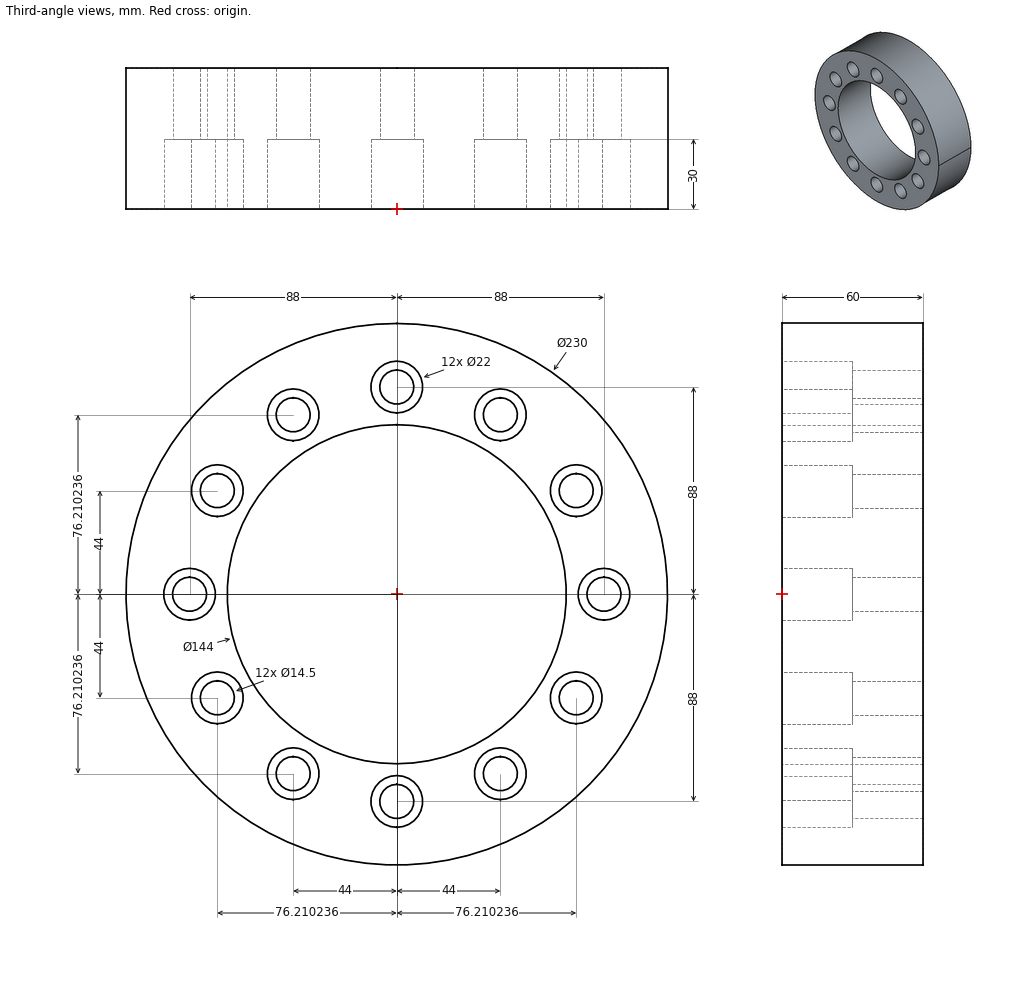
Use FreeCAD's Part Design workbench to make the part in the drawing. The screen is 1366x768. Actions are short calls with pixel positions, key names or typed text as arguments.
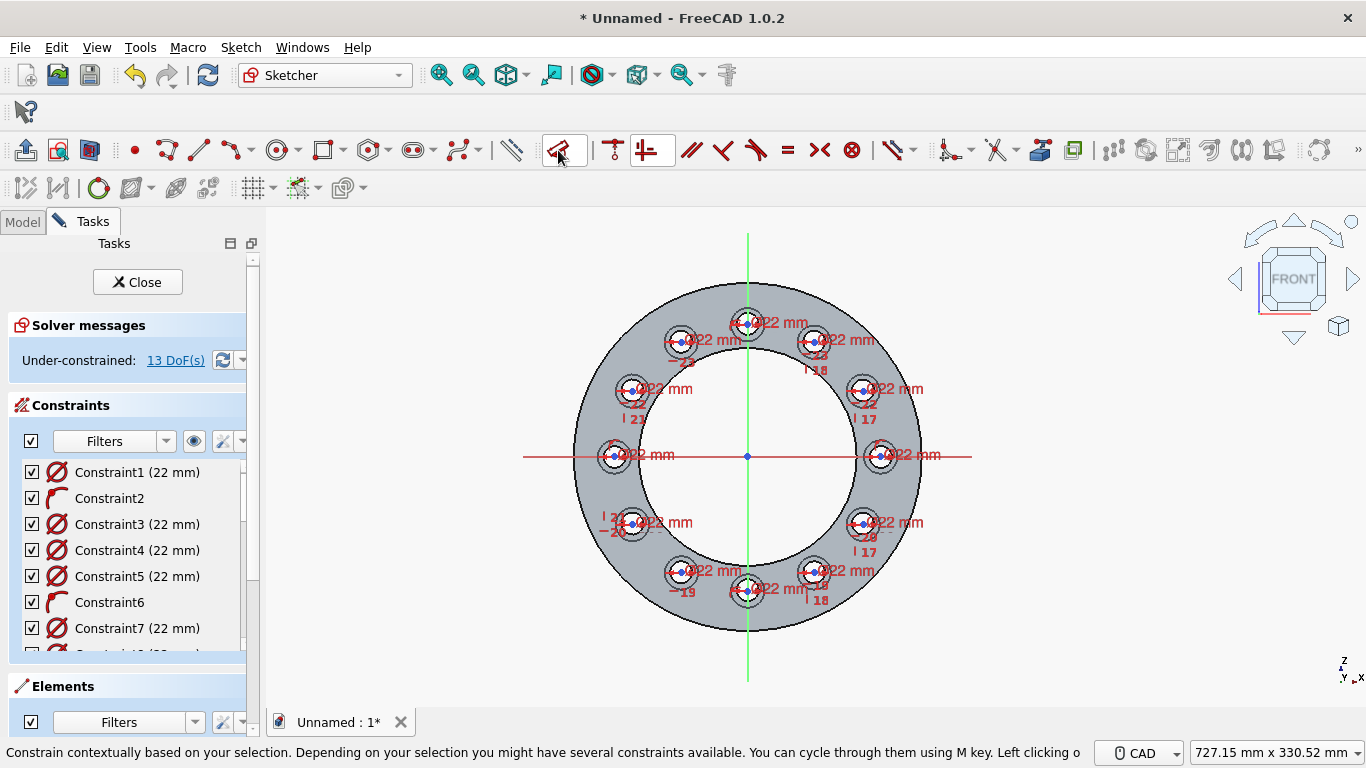
click(748, 325)
click(782, 391)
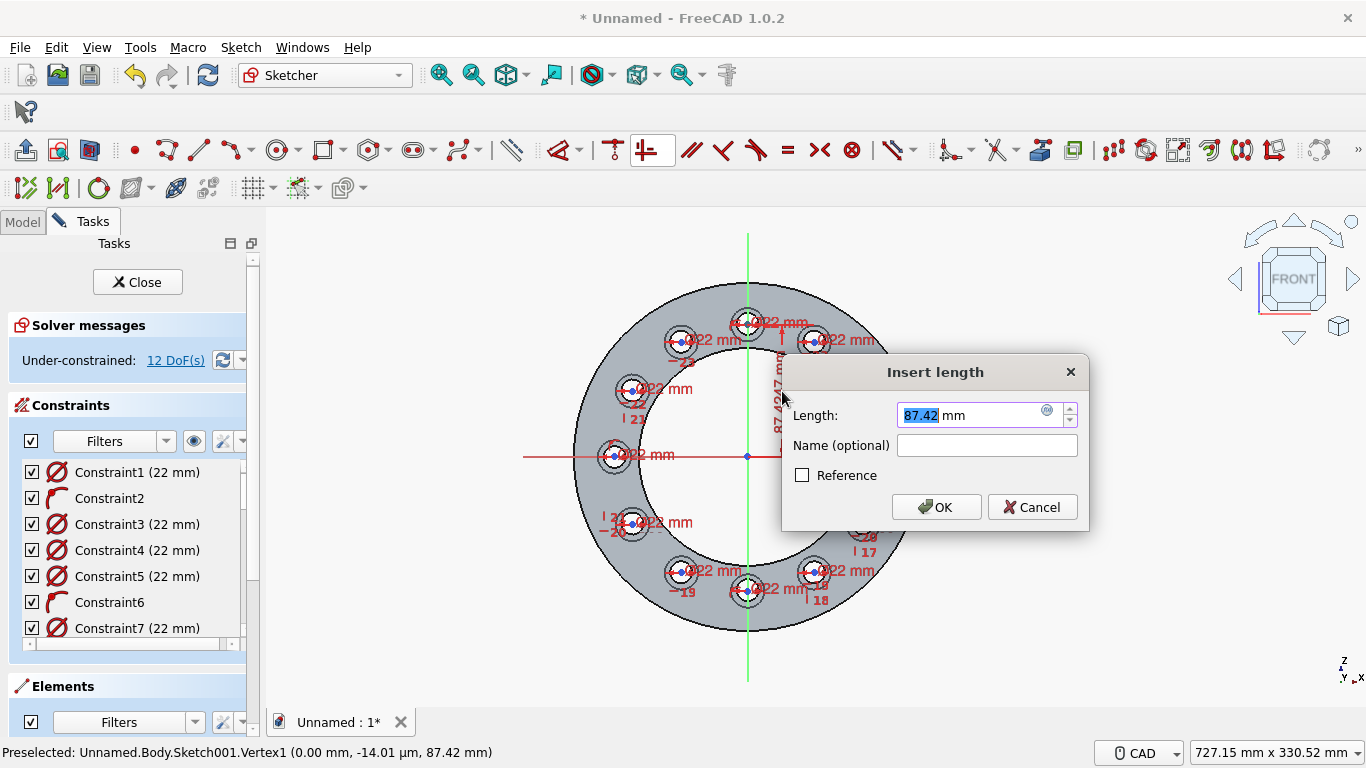
text(88)
key(Return)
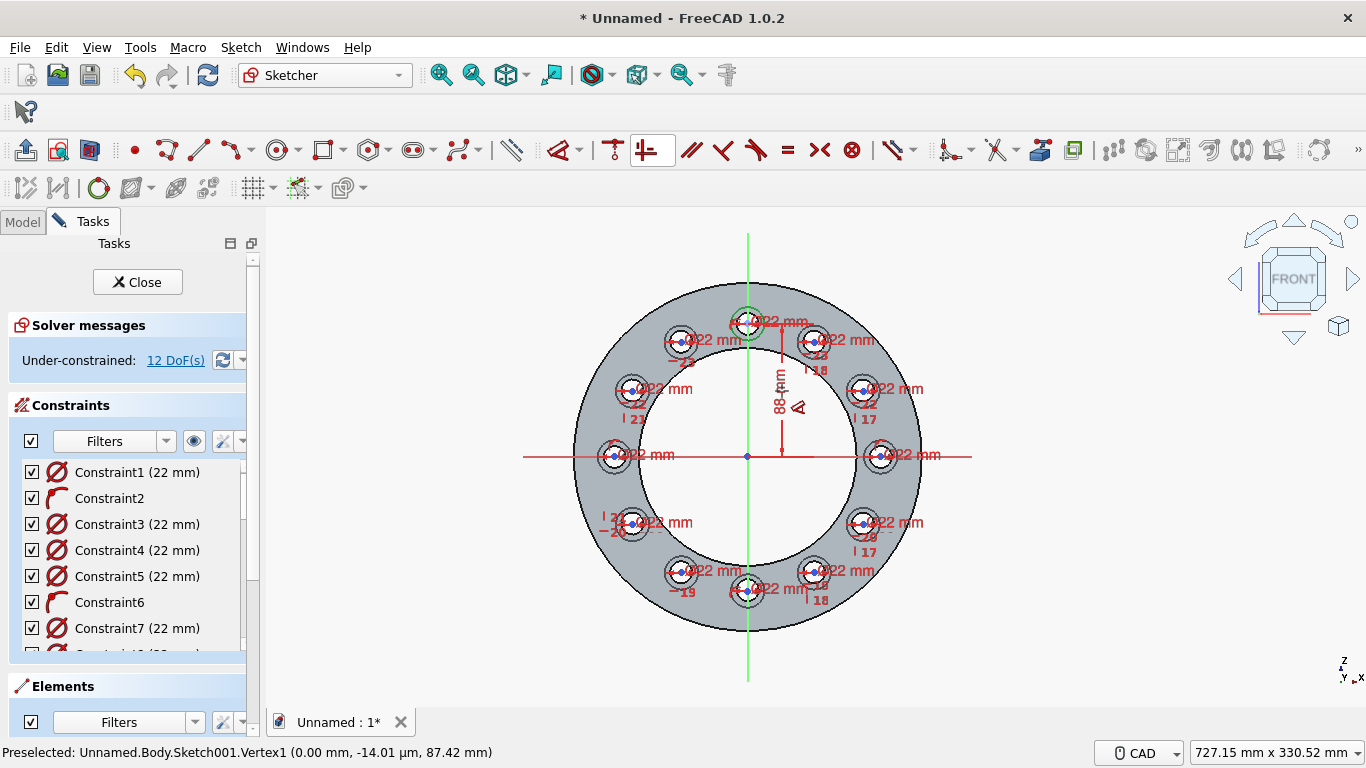
click(814, 342)
click(781, 308)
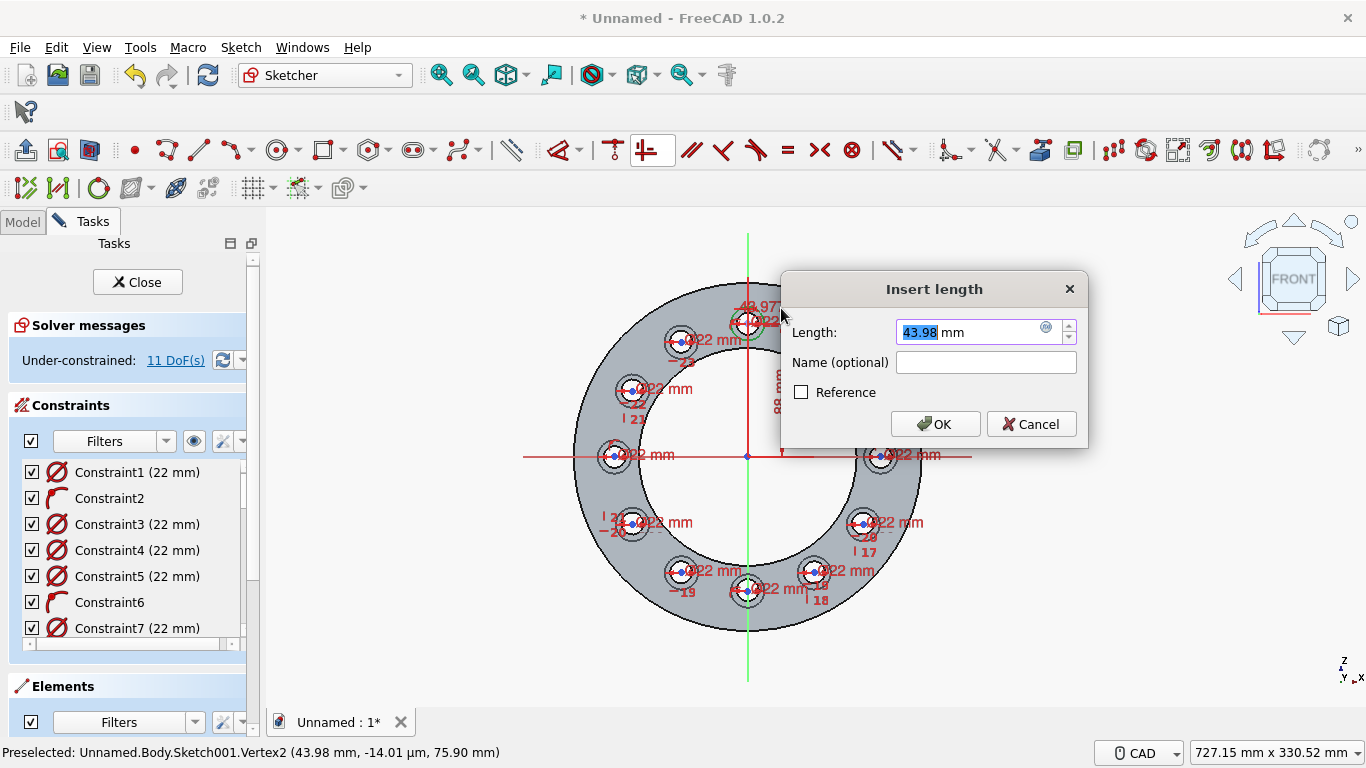
text(44)
key(Return)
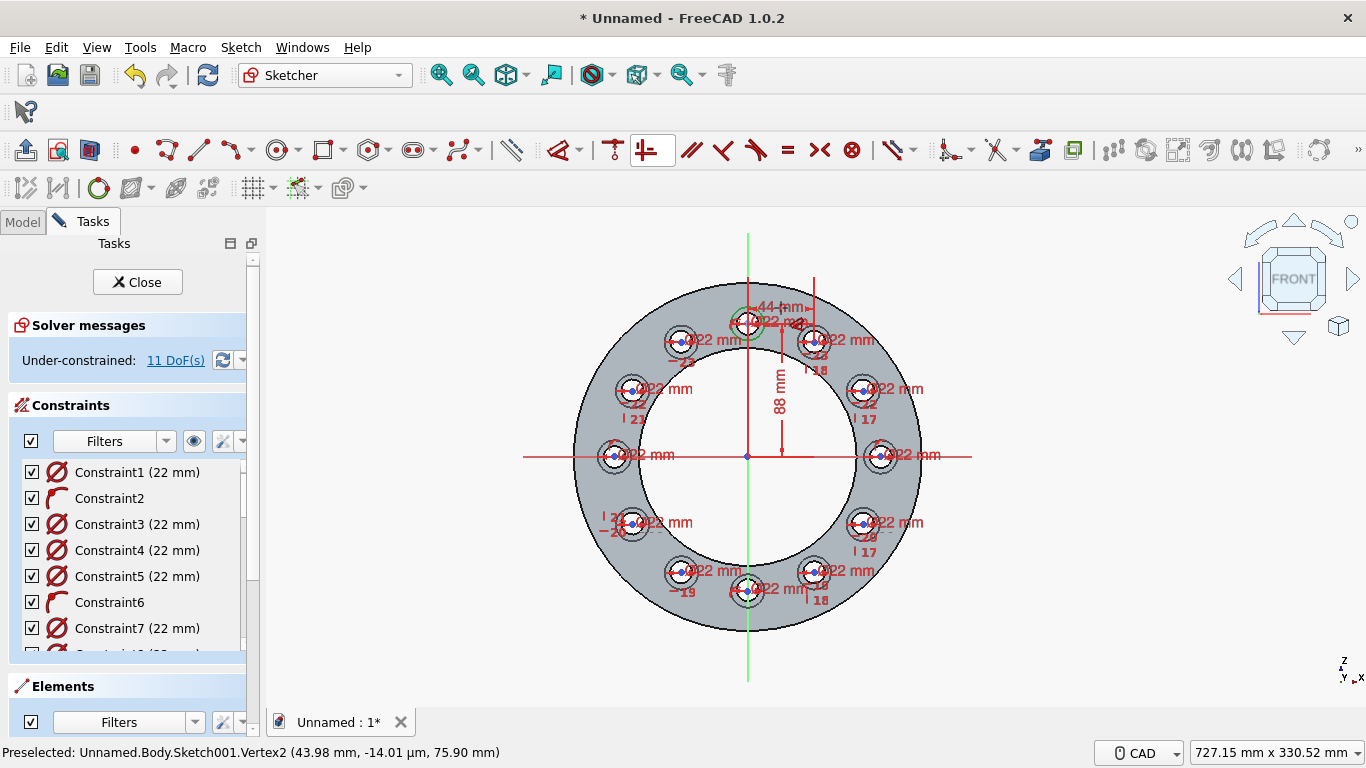
click(863, 391)
click(897, 424)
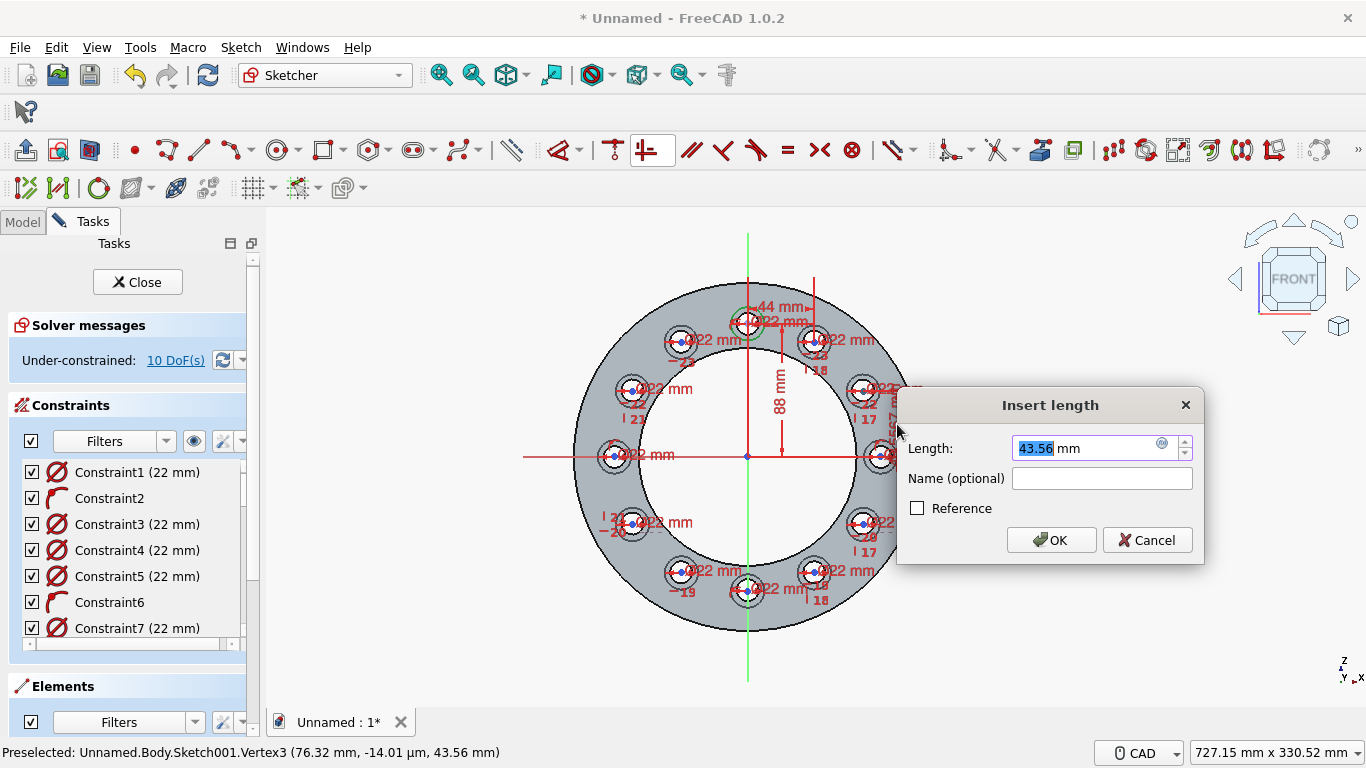
text(44)
key(Return)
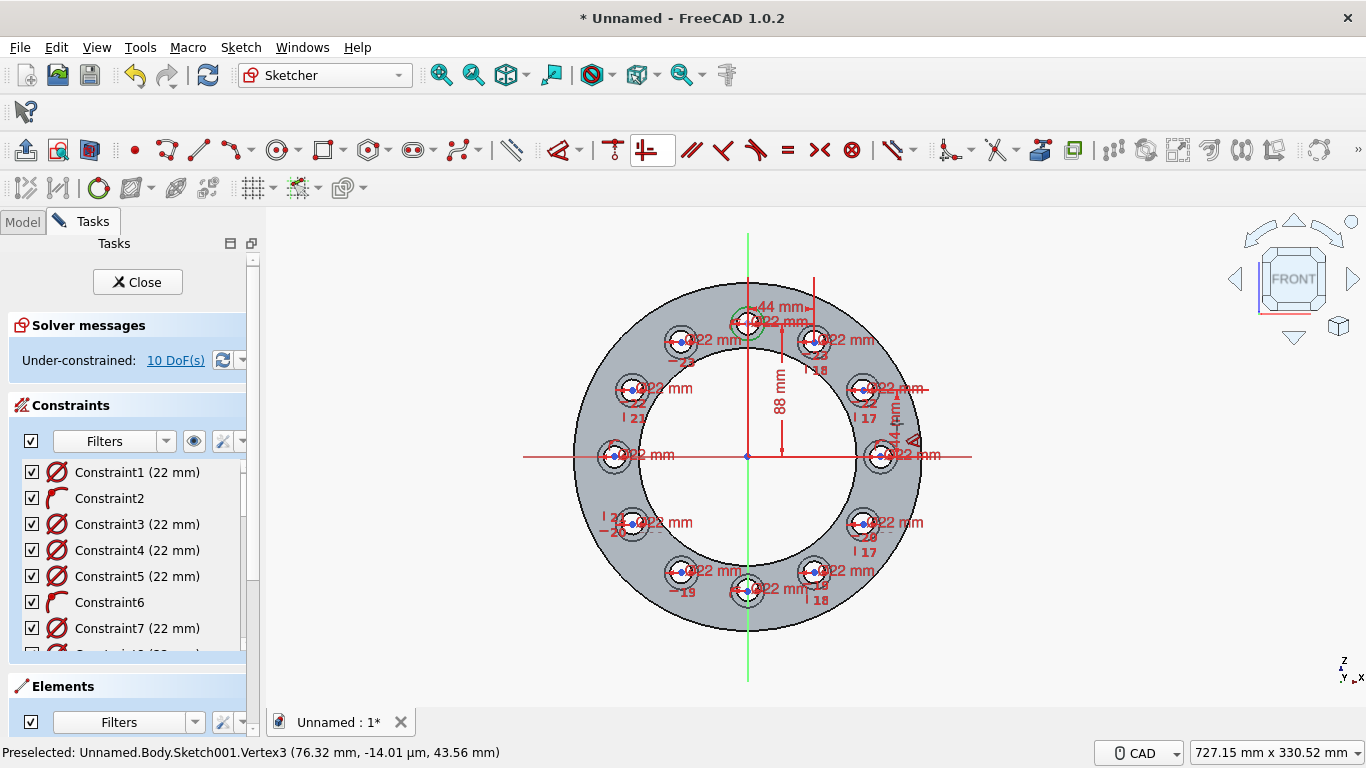
click(881, 457)
click(814, 491)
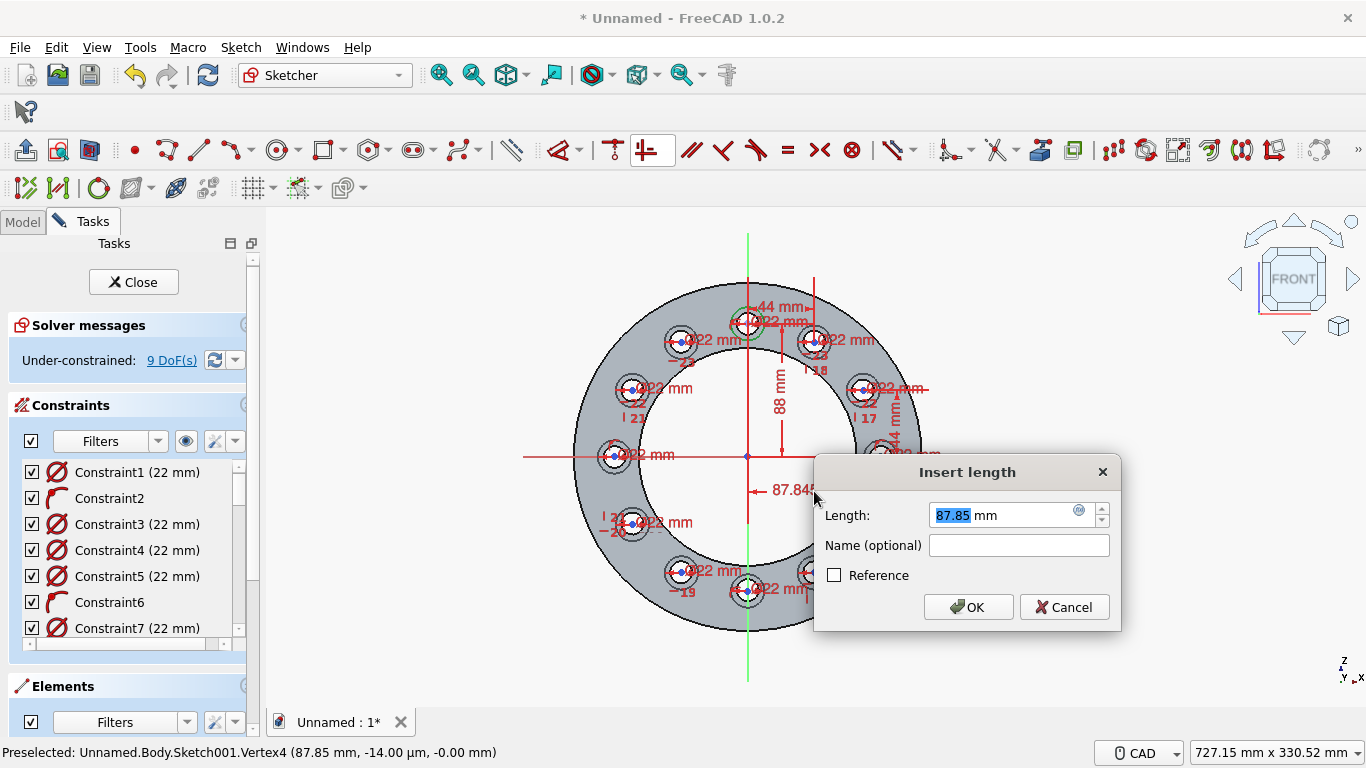
text(88)
key(Return)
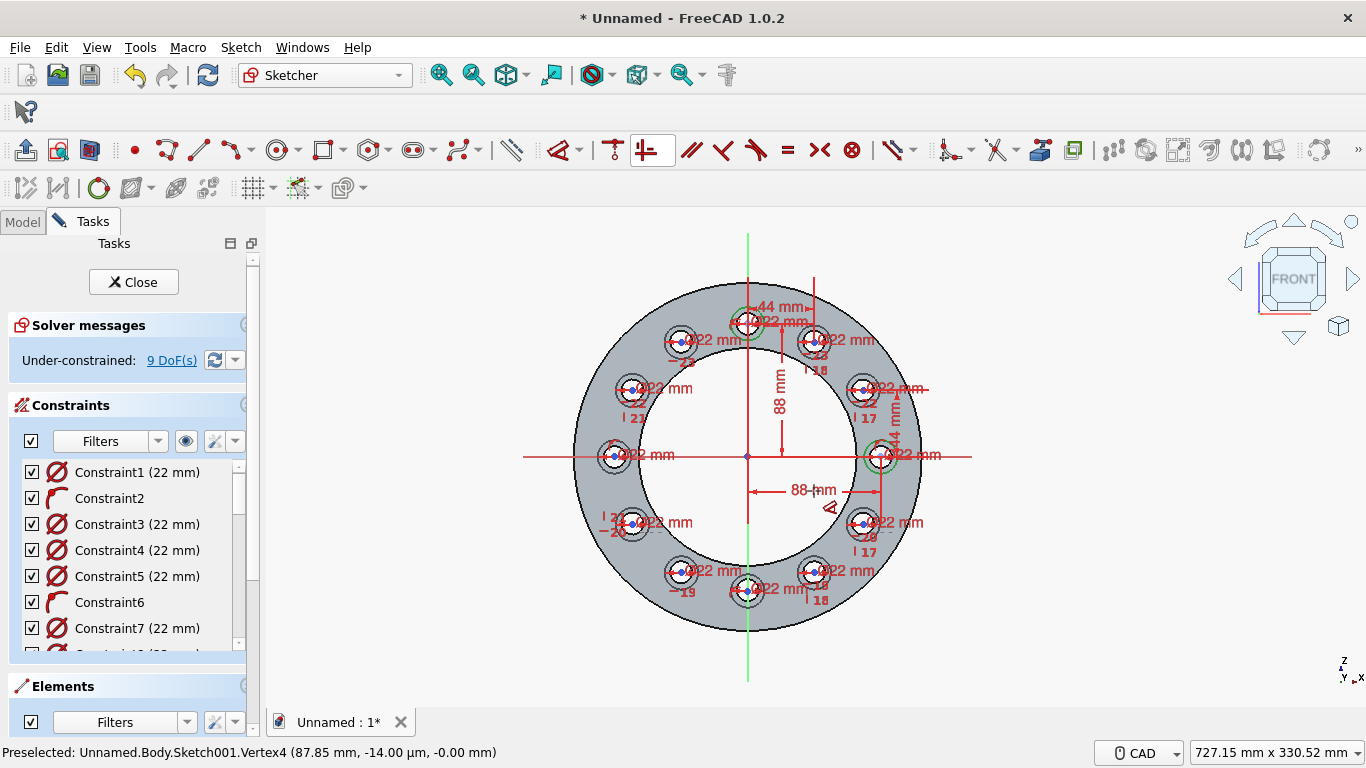
click(863, 525)
click(897, 491)